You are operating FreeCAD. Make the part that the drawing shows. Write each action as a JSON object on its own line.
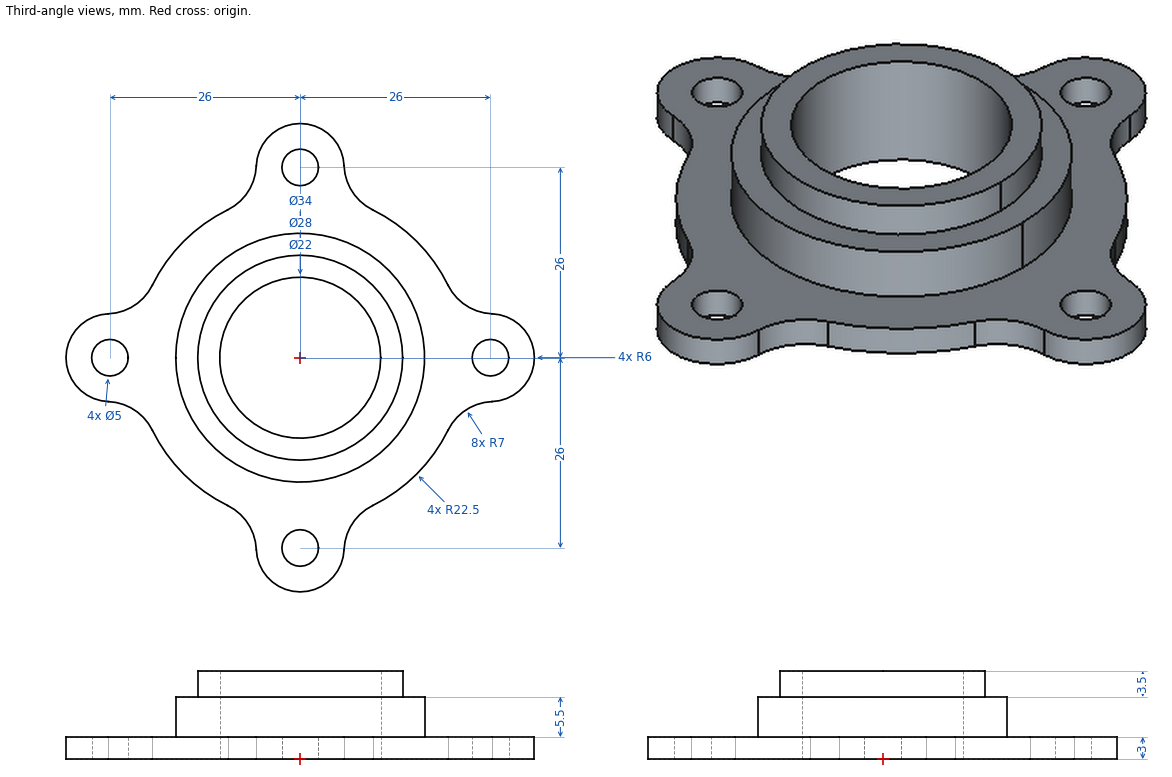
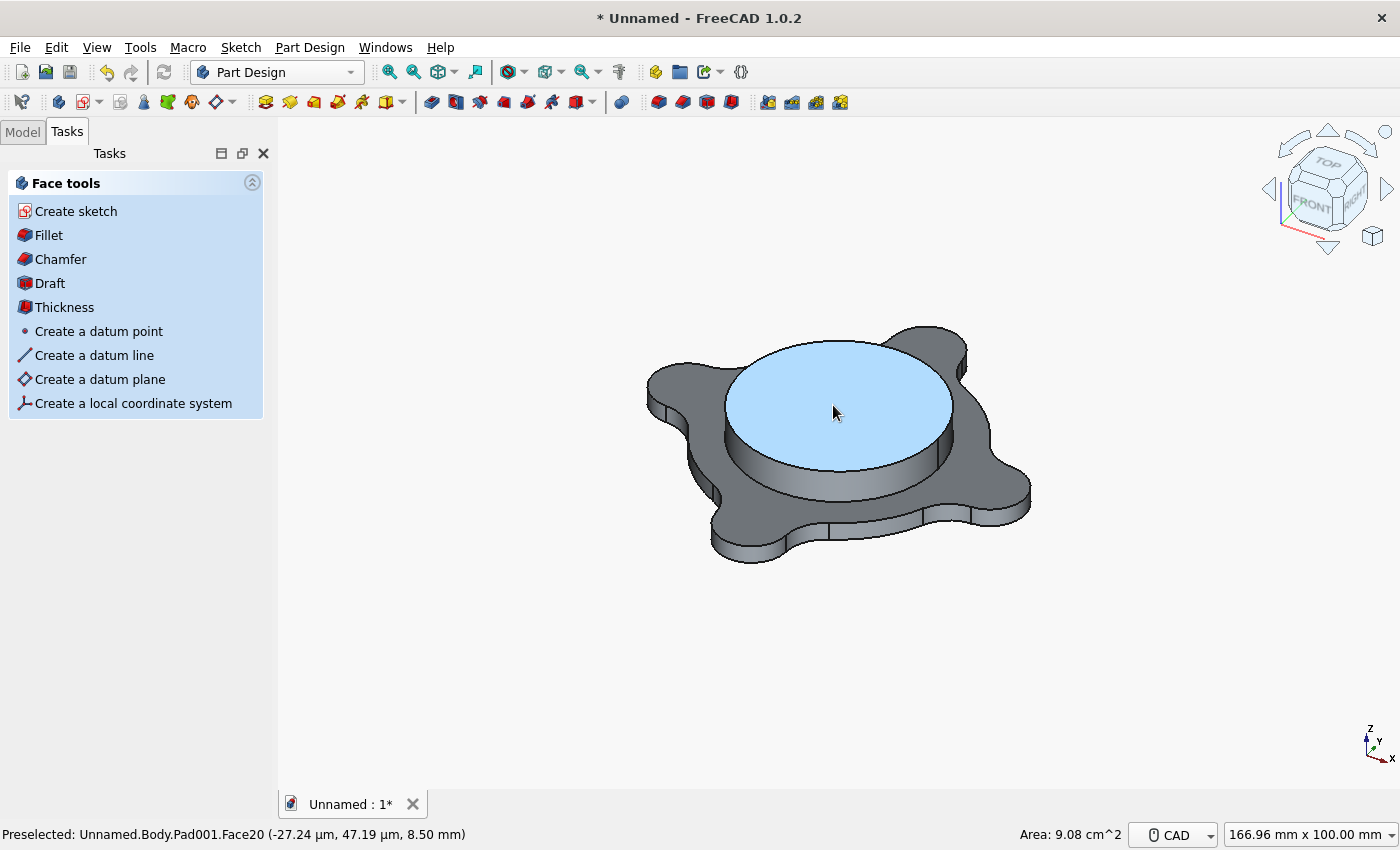
{"action": "left_click", "coordinate": [84, 102]}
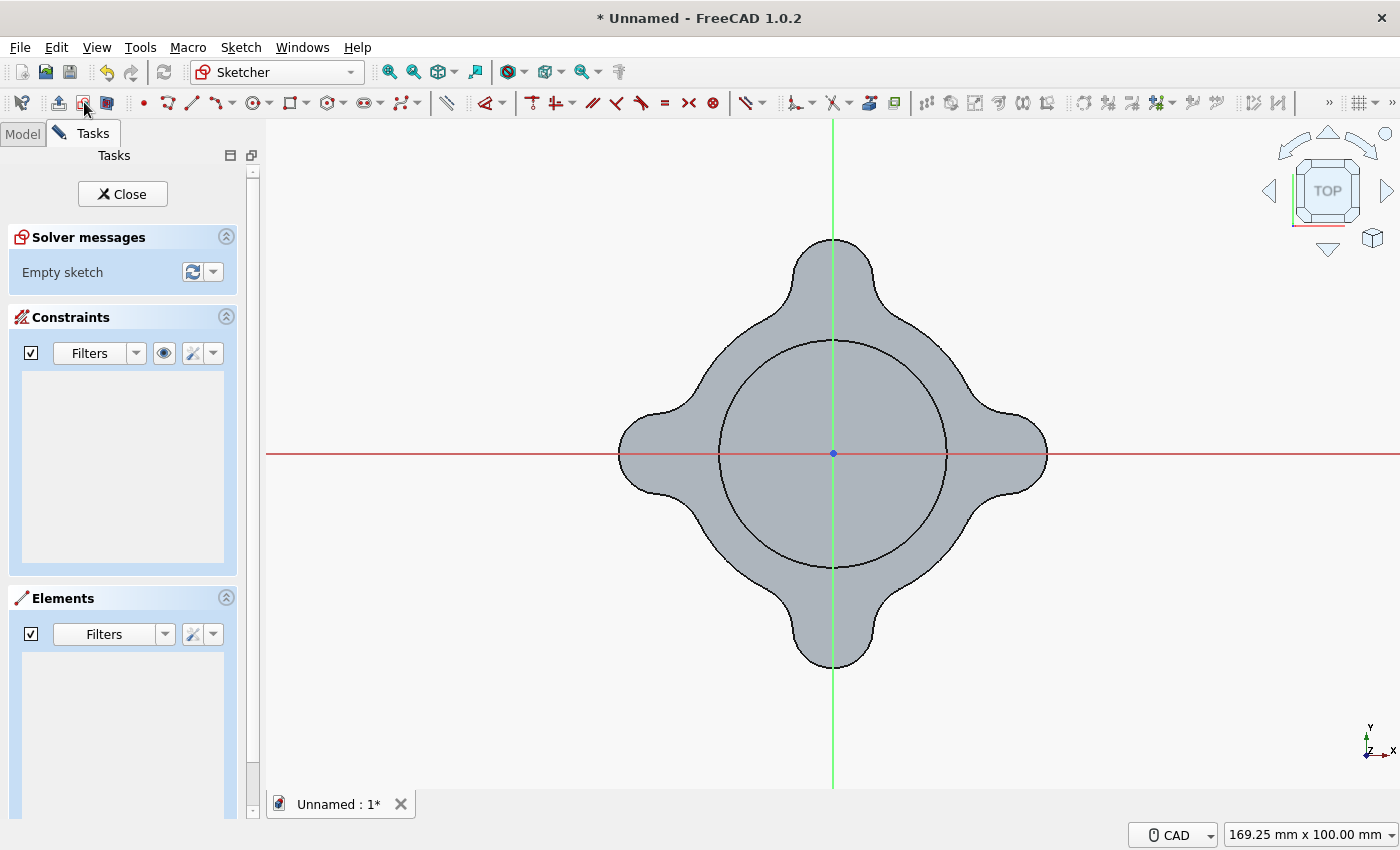
{"action": "scroll", "coordinate": [889, 454], "scroll_direction": "up", "scroll_amount": 4}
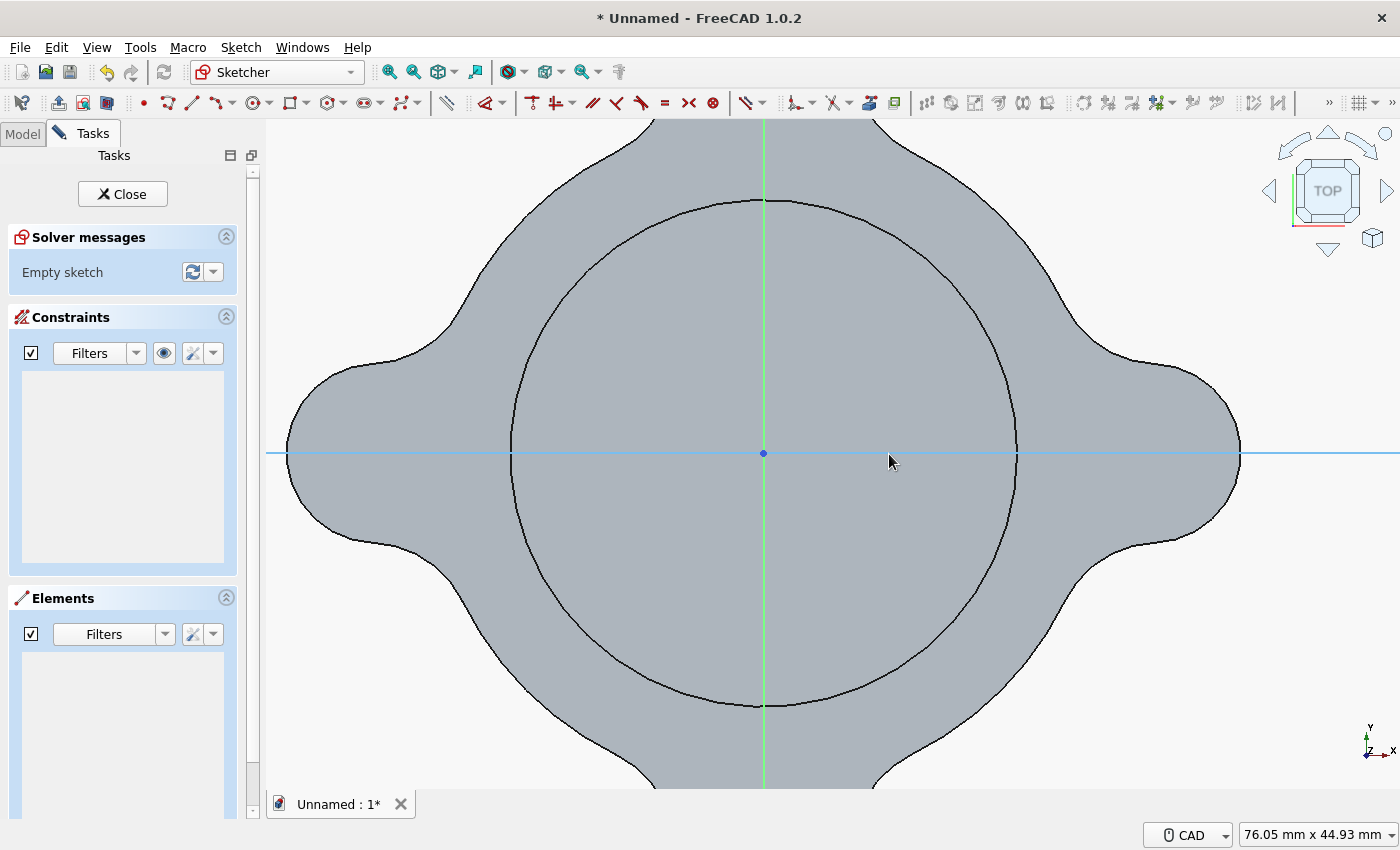
{"action": "left_click", "coordinate": [254, 104]}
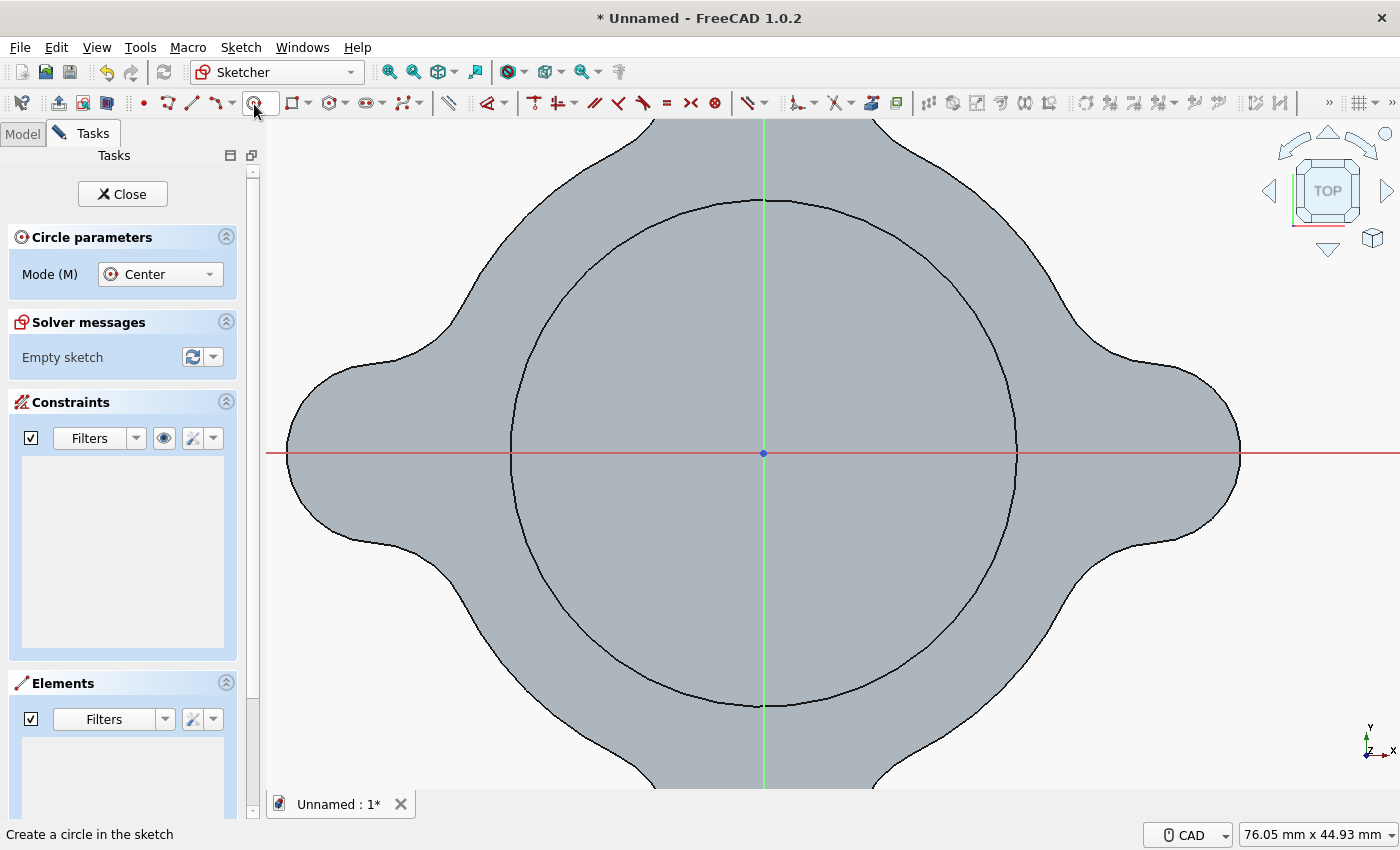
{"action": "left_click", "coordinate": [764, 453]}
{"action": "mouse_move", "coordinate": [911, 306]}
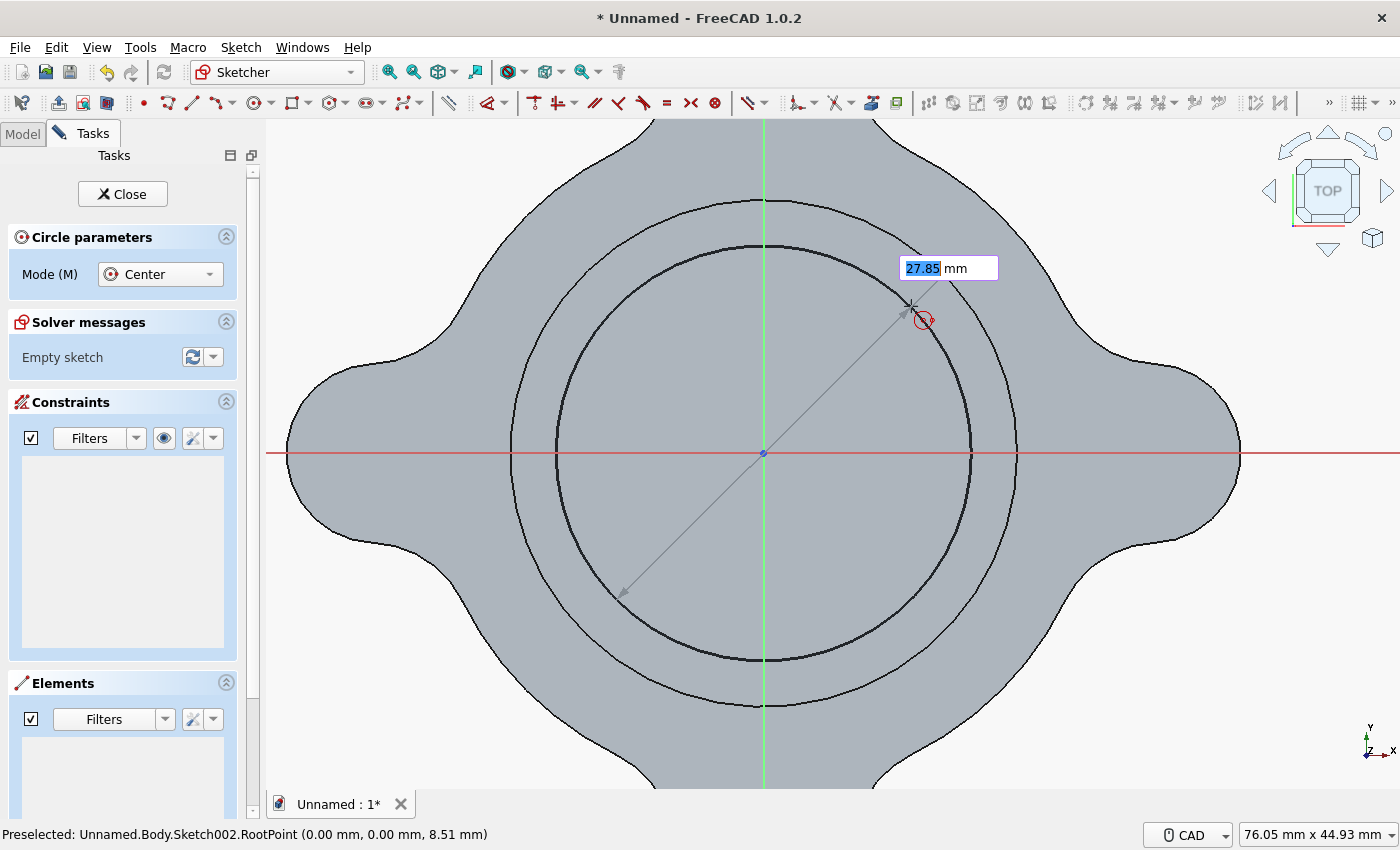
{"action": "type", "text": "28"}
{"action": "key", "text": "Return"}
{"action": "key", "text": "Escape"}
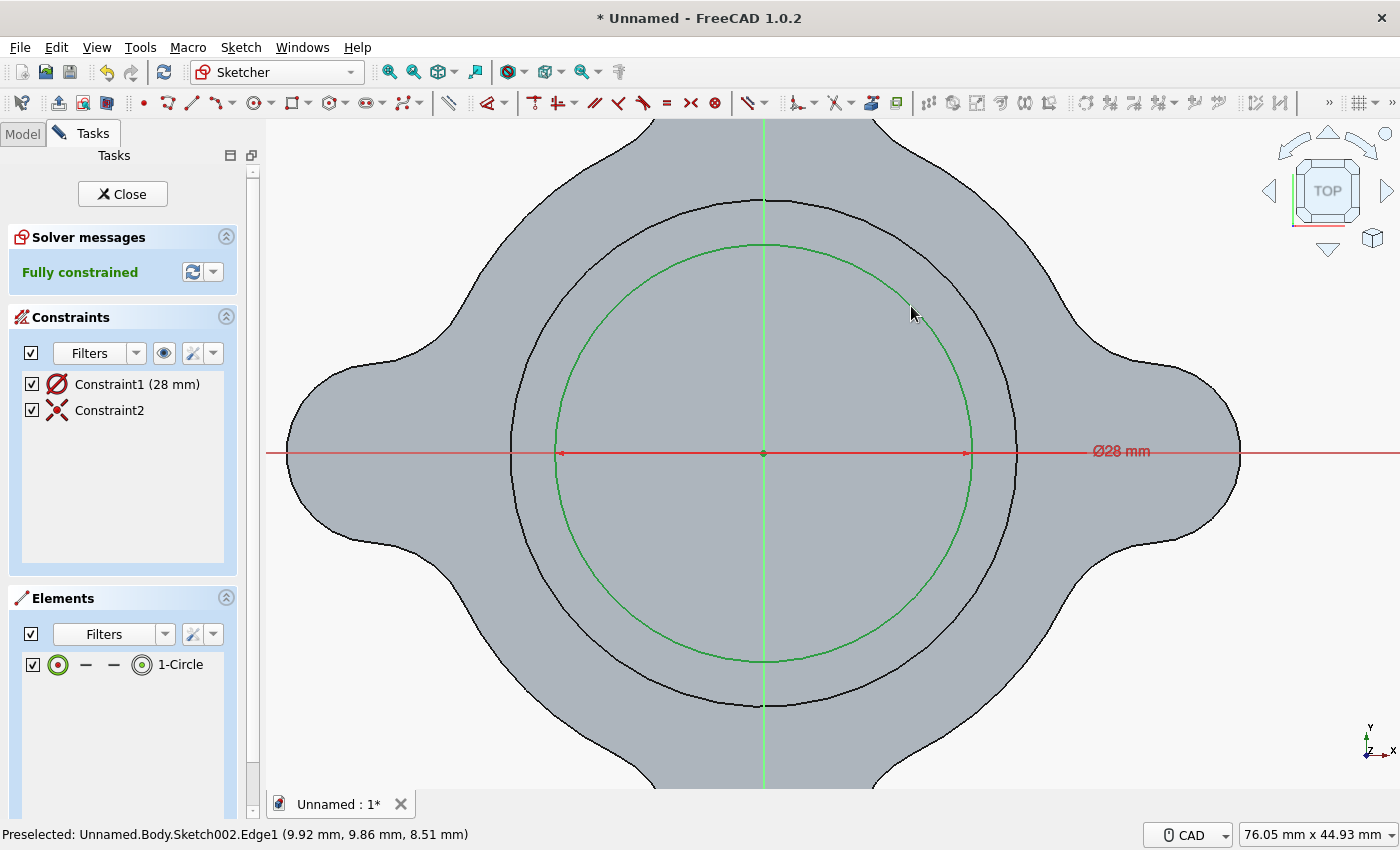
{"action": "left_click", "coordinate": [123, 194]}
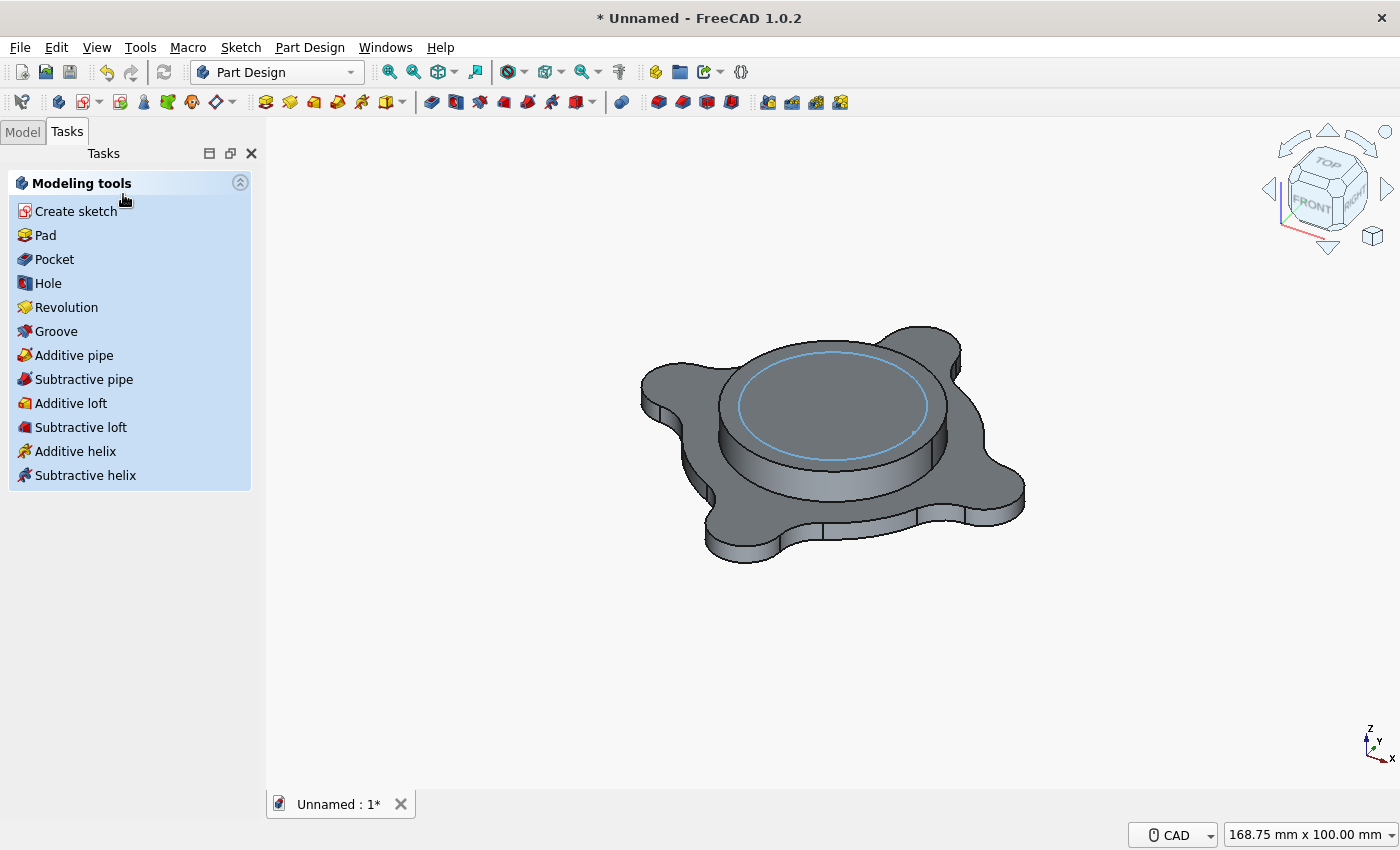
{"action": "left_click", "coordinate": [266, 102]}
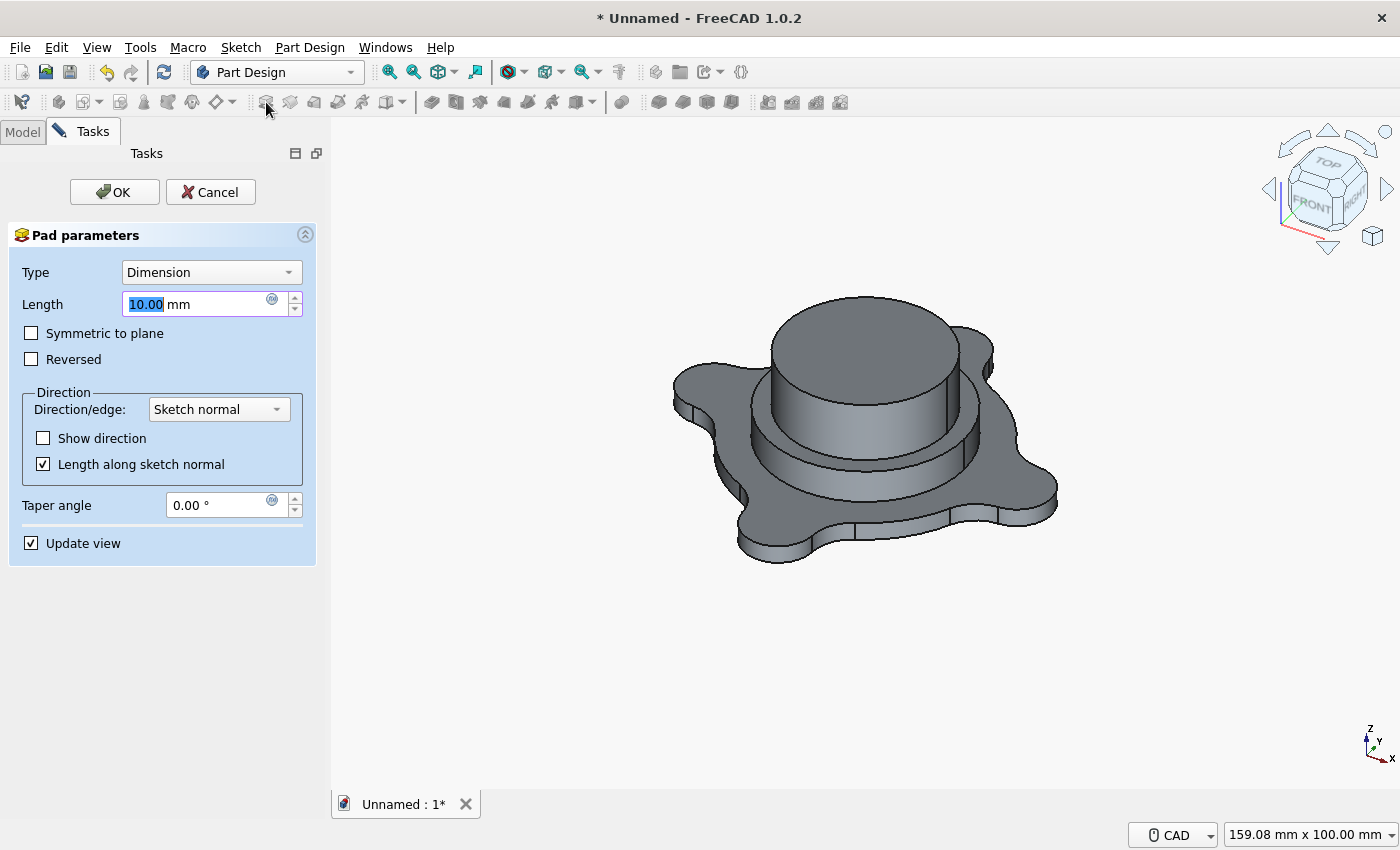
{"action": "type", "text": "3.5"}
{"action": "key", "text": "Tab"}